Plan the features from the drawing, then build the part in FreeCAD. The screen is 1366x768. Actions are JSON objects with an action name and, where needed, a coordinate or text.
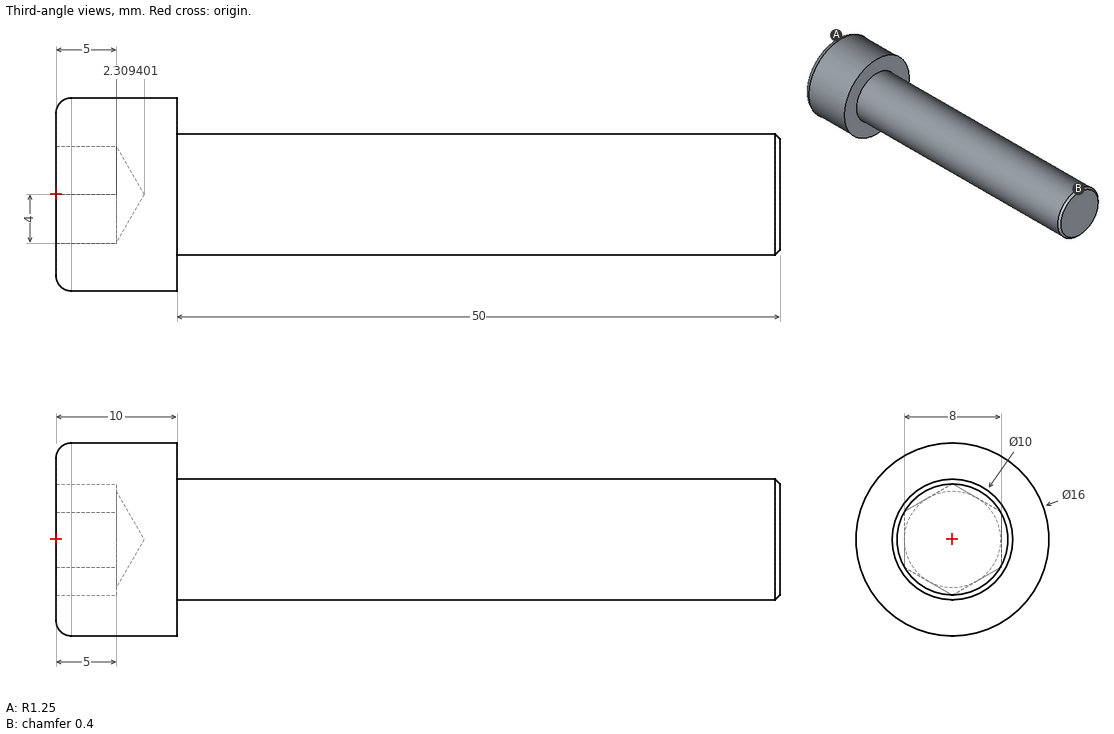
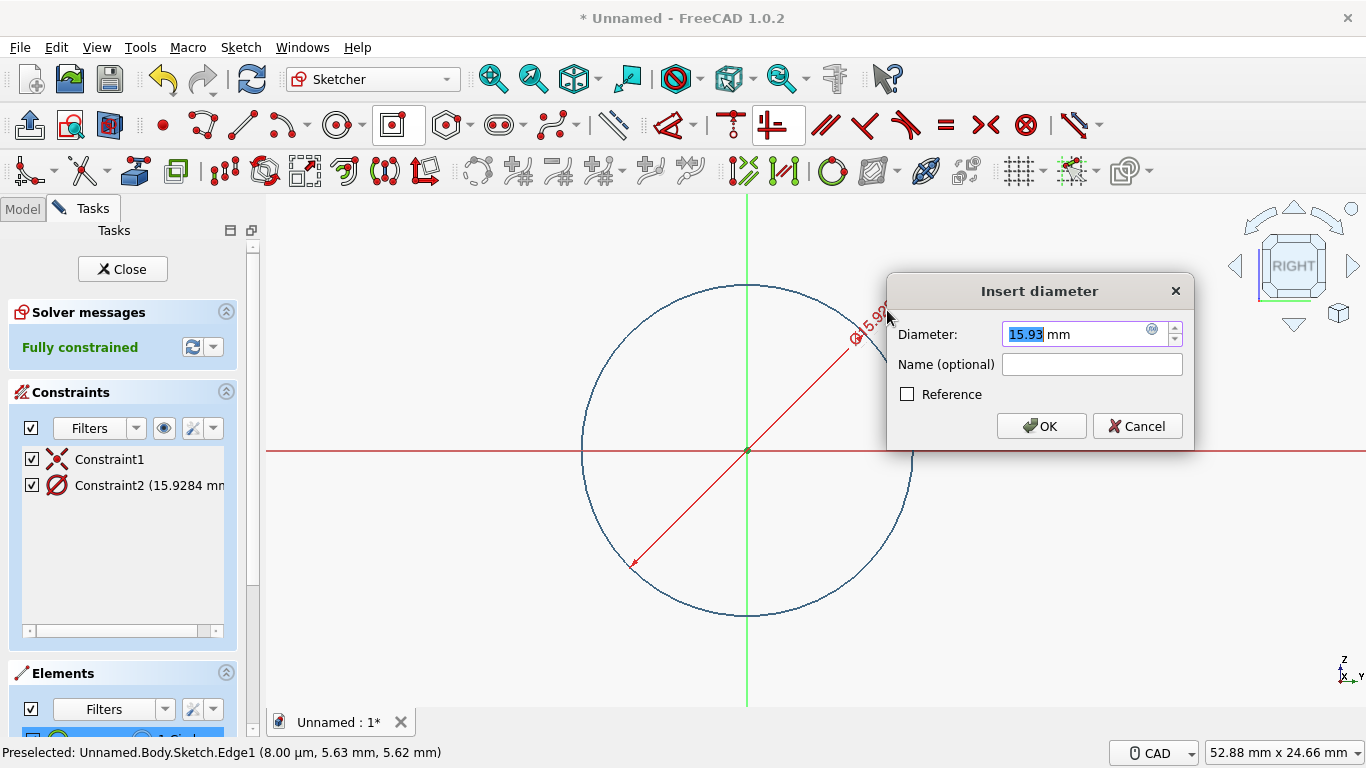
{"action": "type", "text": "16"}
{"action": "key", "text": "Return"}
{"action": "key", "text": "Escape"}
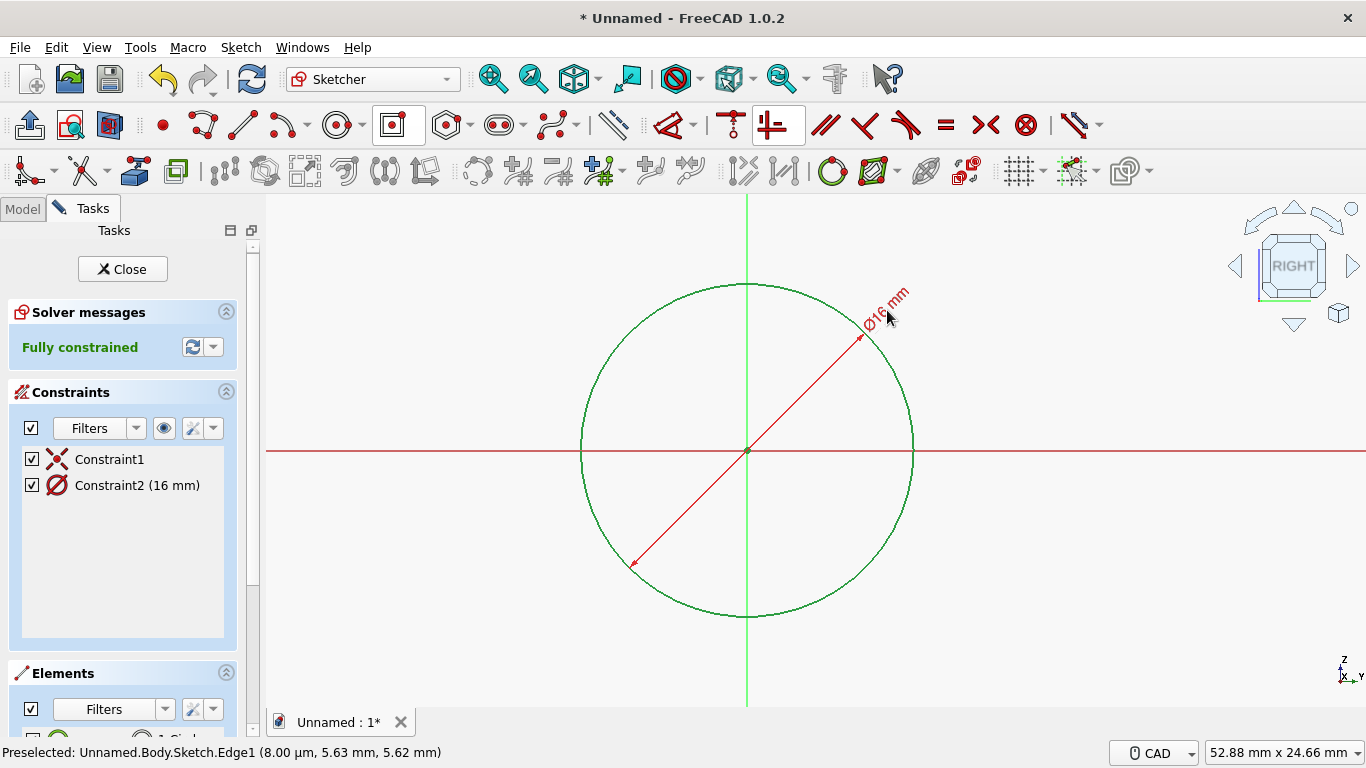
{"action": "left_click", "coordinate": [123, 269]}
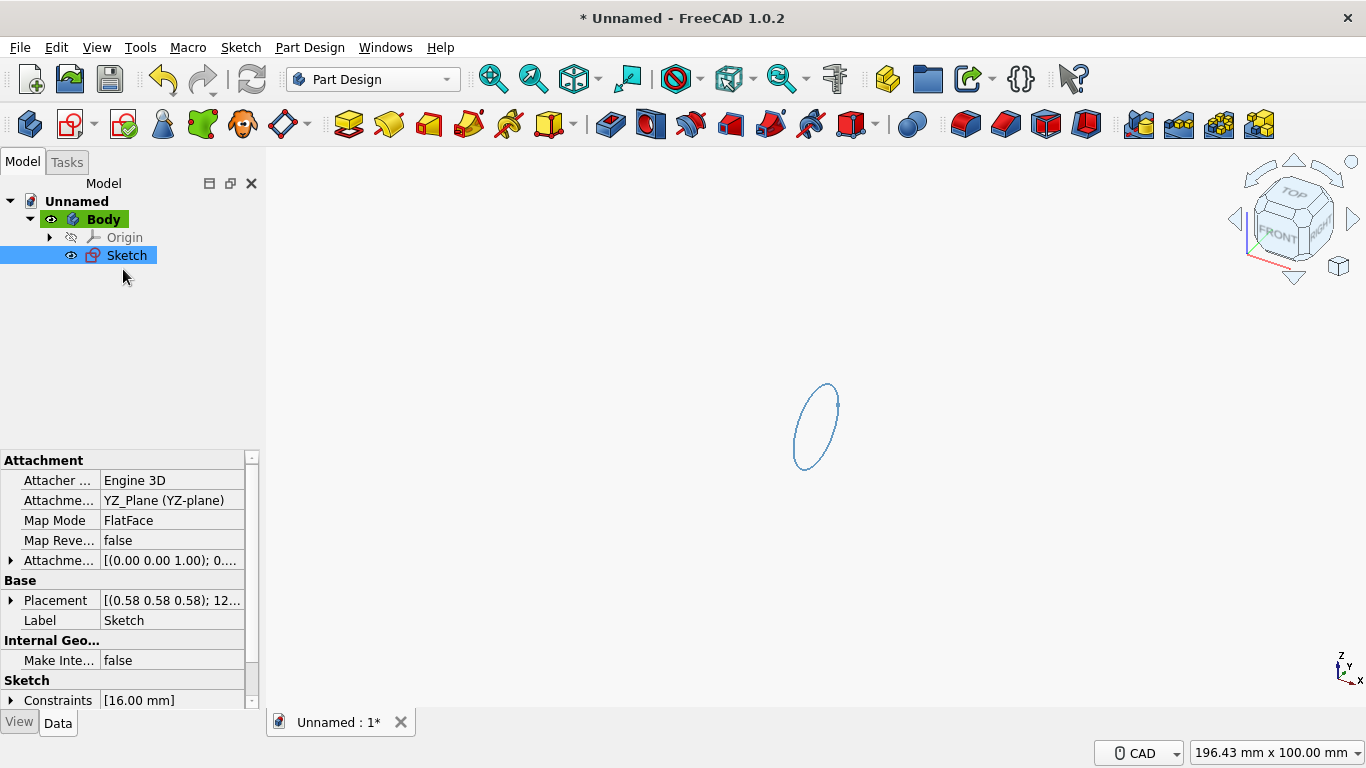
{"action": "left_click", "coordinate": [350, 124]}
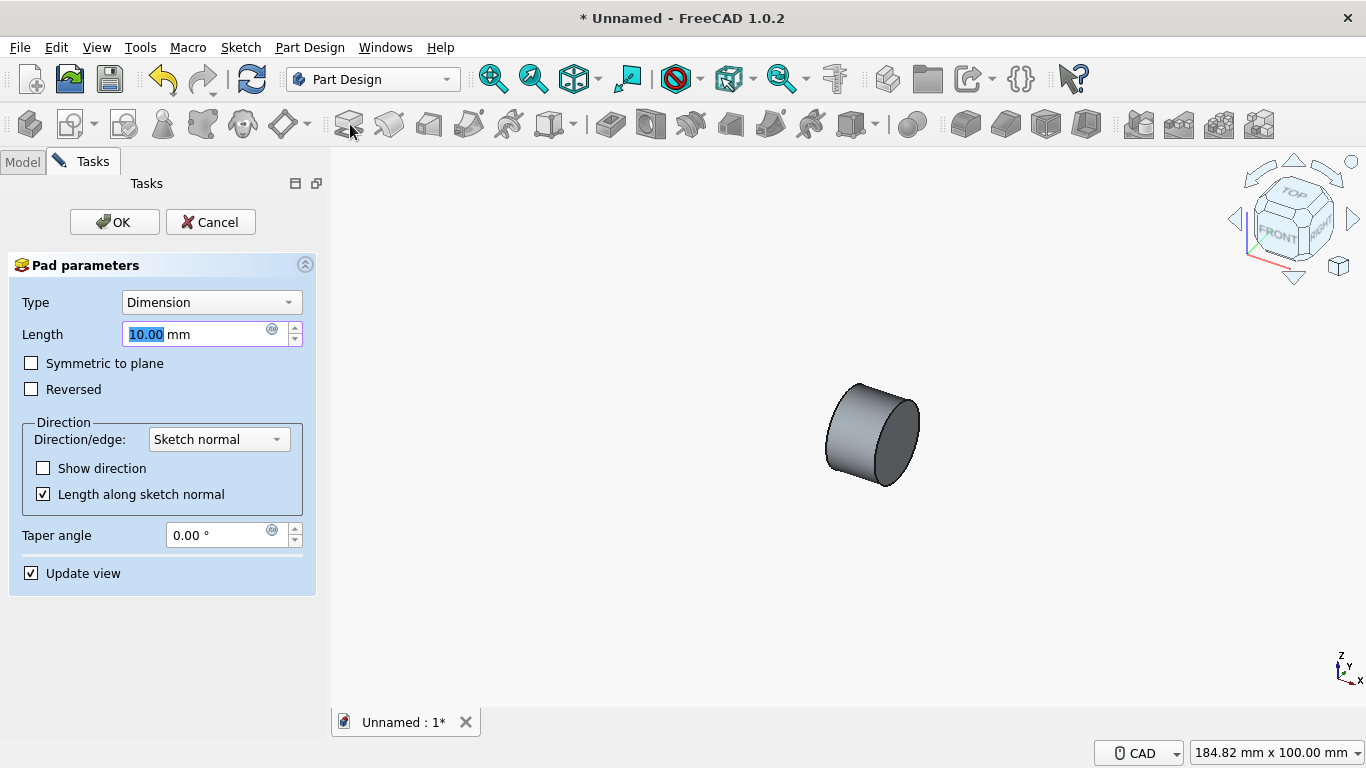
{"action": "type", "text": "10"}
{"action": "key", "text": "Tab"}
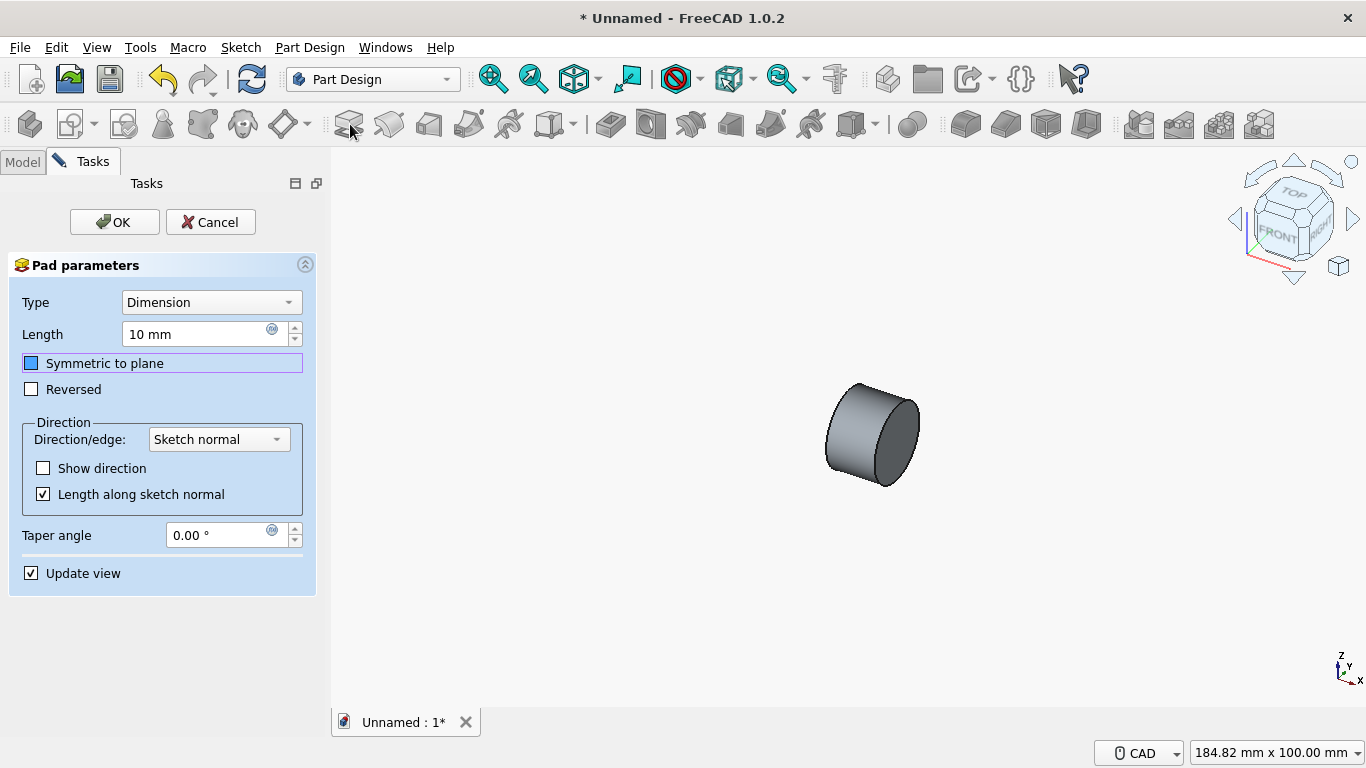
{"action": "left_click", "coordinate": [115, 222]}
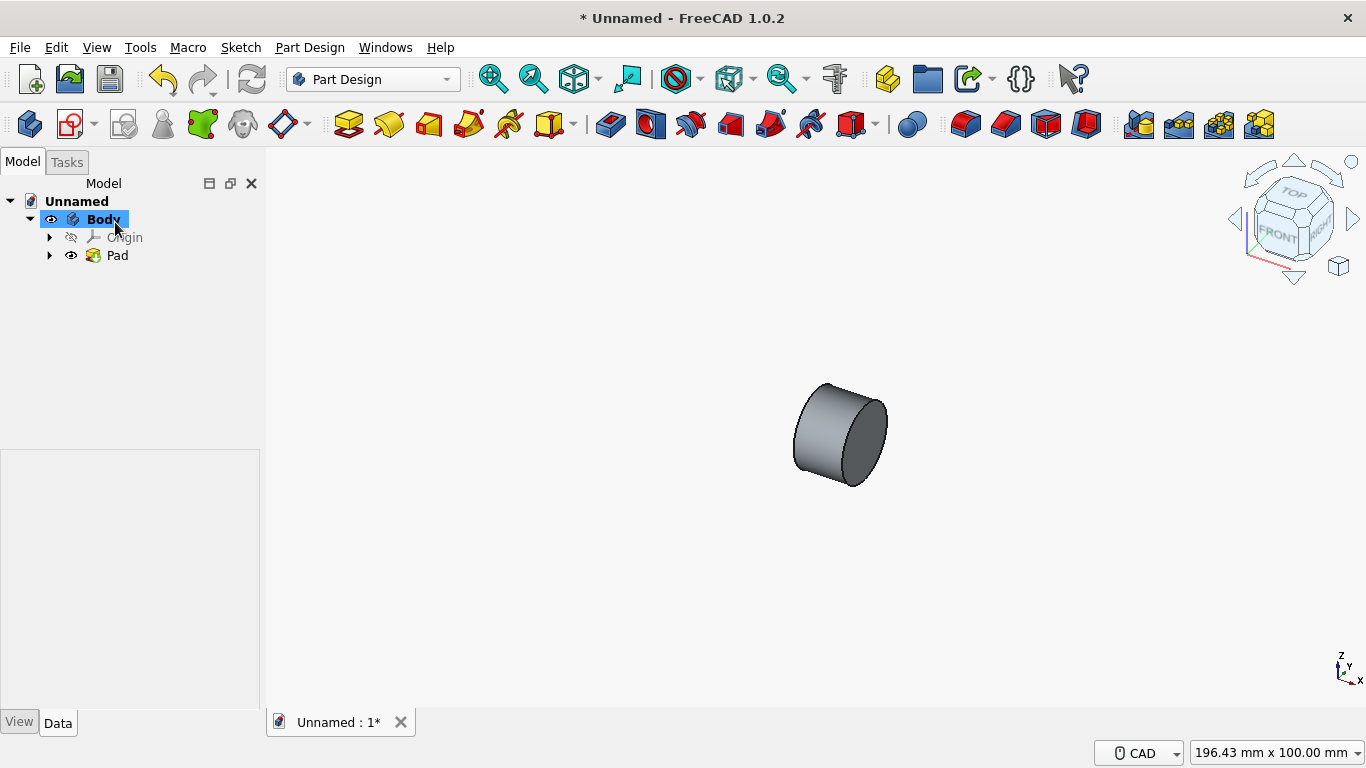
{"action": "left_click", "coordinate": [494, 80]}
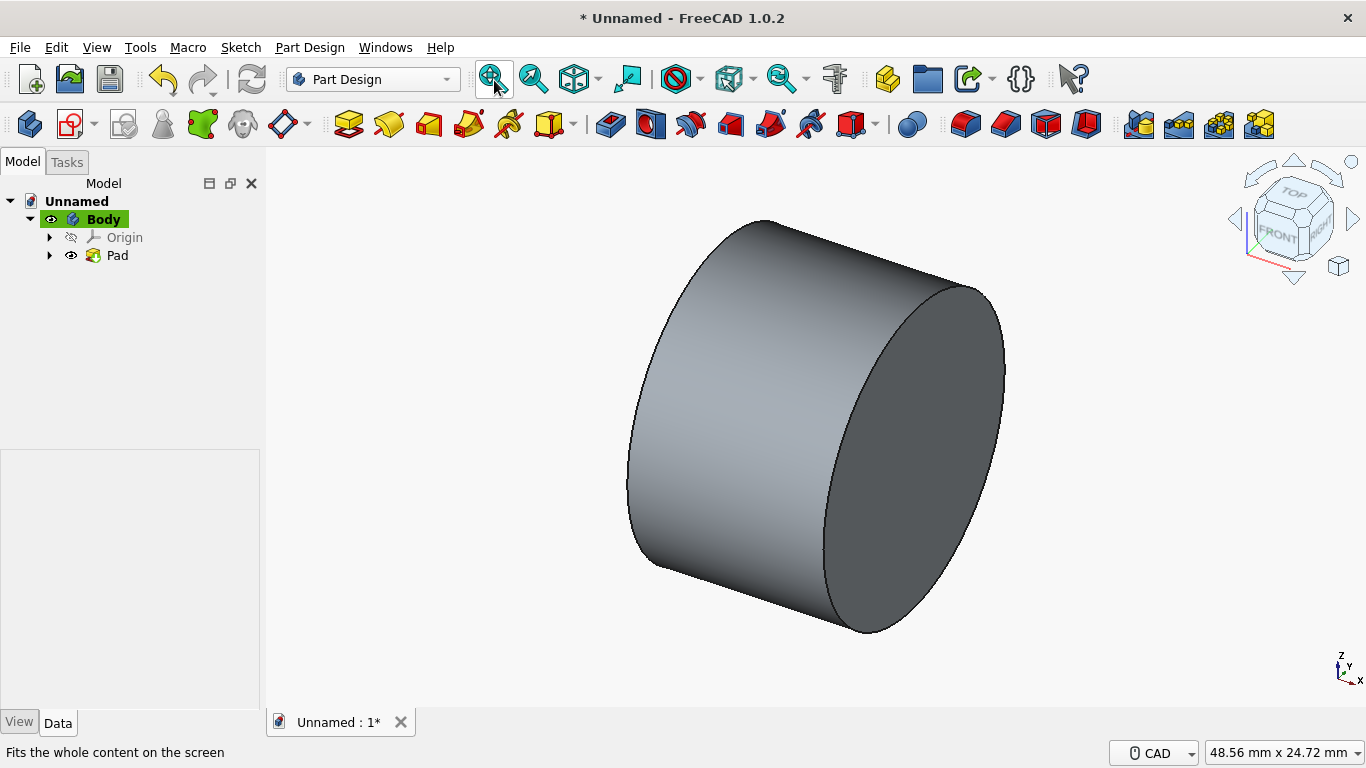
{"action": "left_click", "coordinate": [914, 458]}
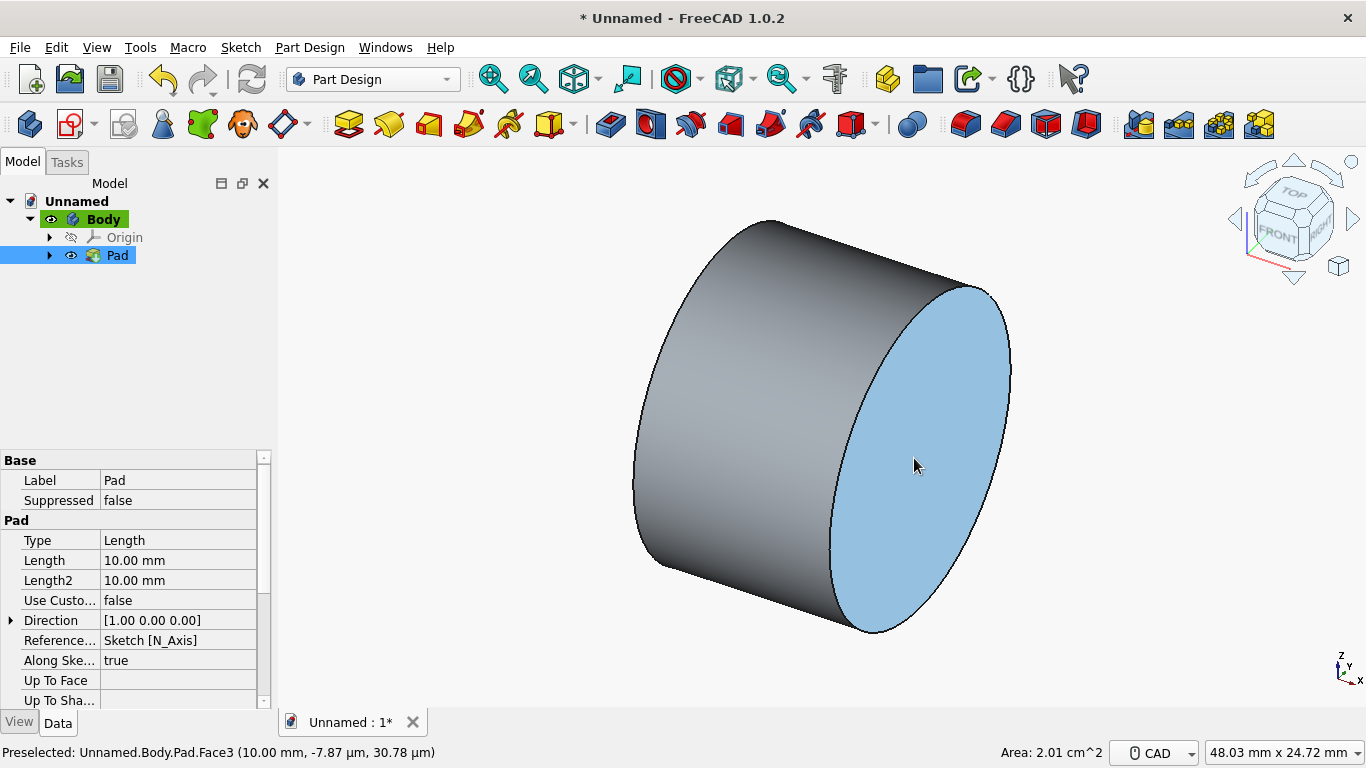
{"action": "left_click", "coordinate": [70, 124]}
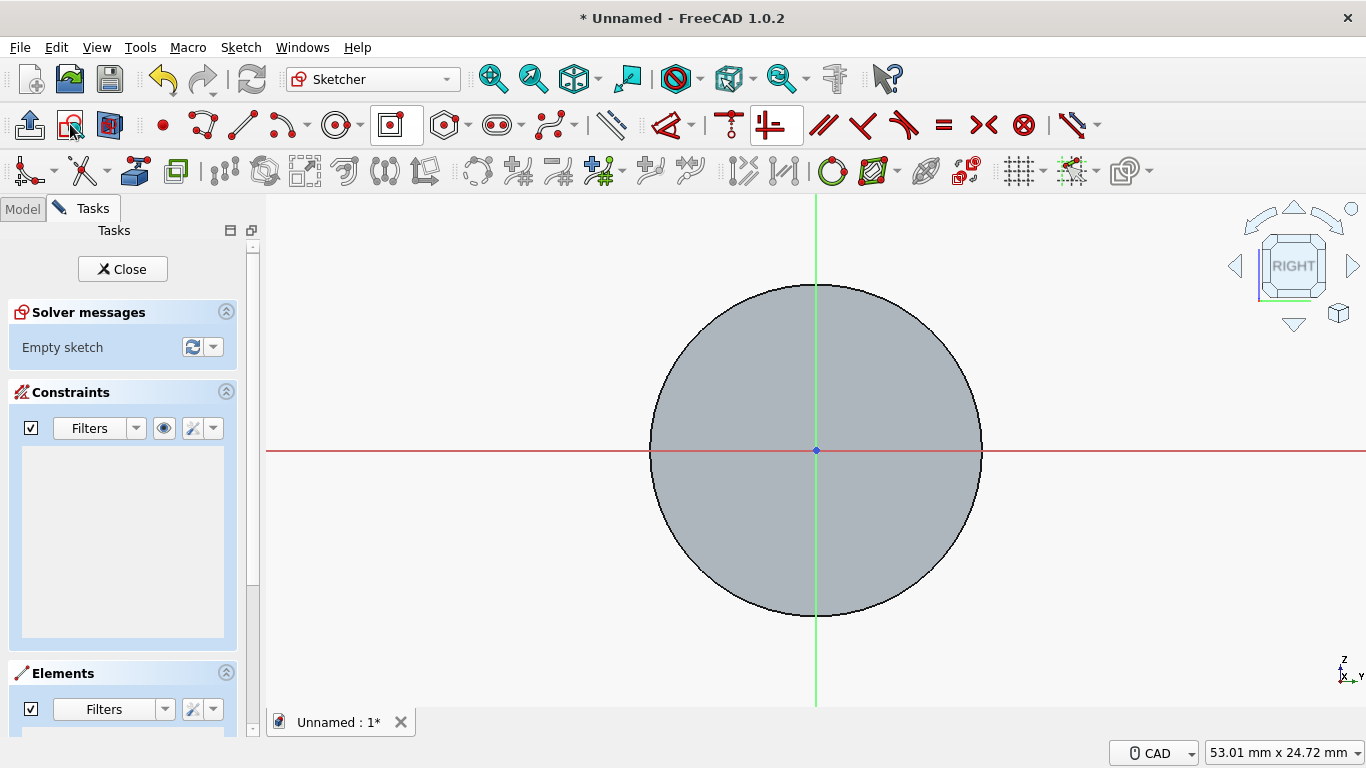
{"action": "scroll", "coordinate": [955, 451], "scroll_direction": "up", "scroll_amount": 2}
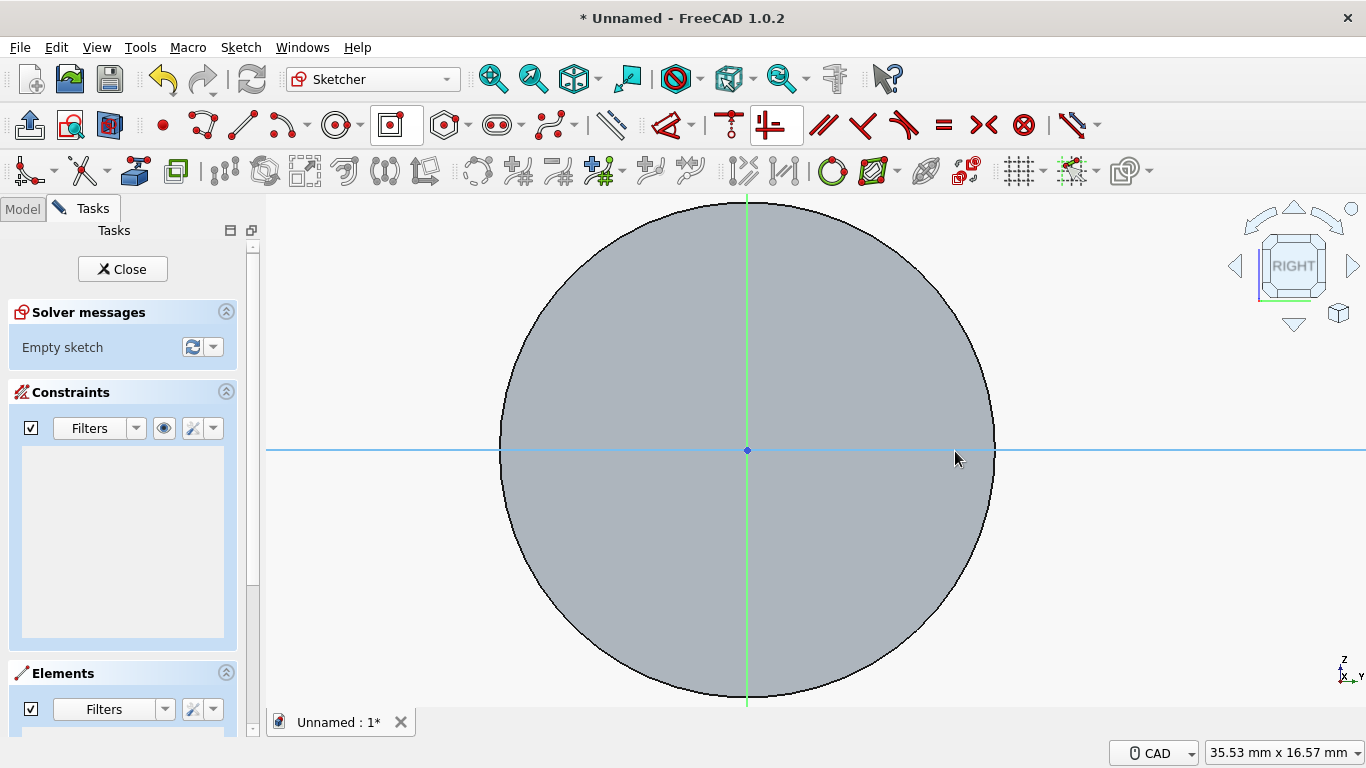
{"action": "left_click", "coordinate": [336, 126]}